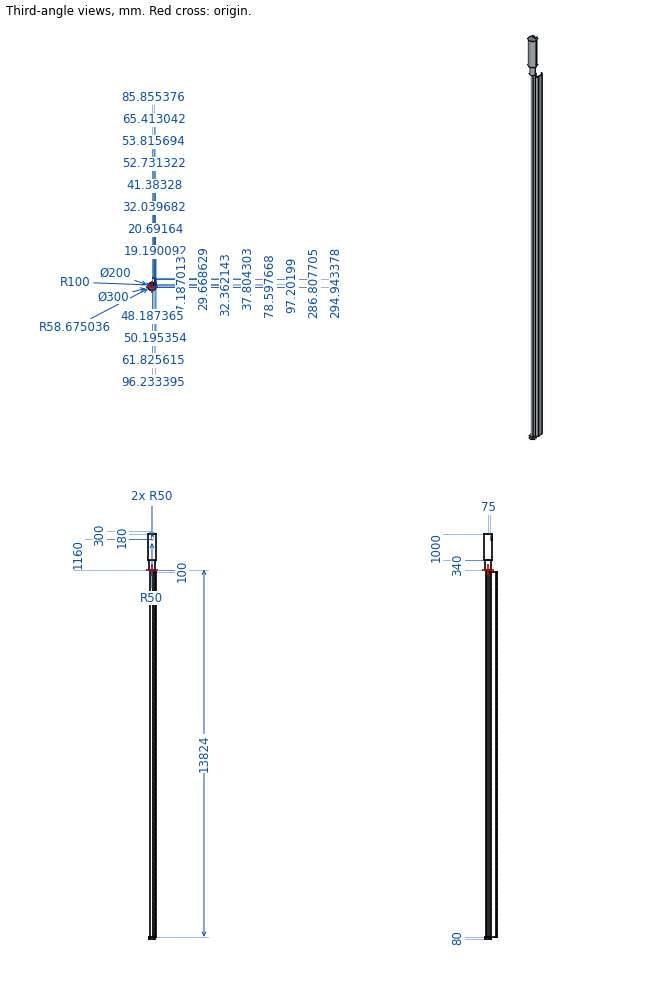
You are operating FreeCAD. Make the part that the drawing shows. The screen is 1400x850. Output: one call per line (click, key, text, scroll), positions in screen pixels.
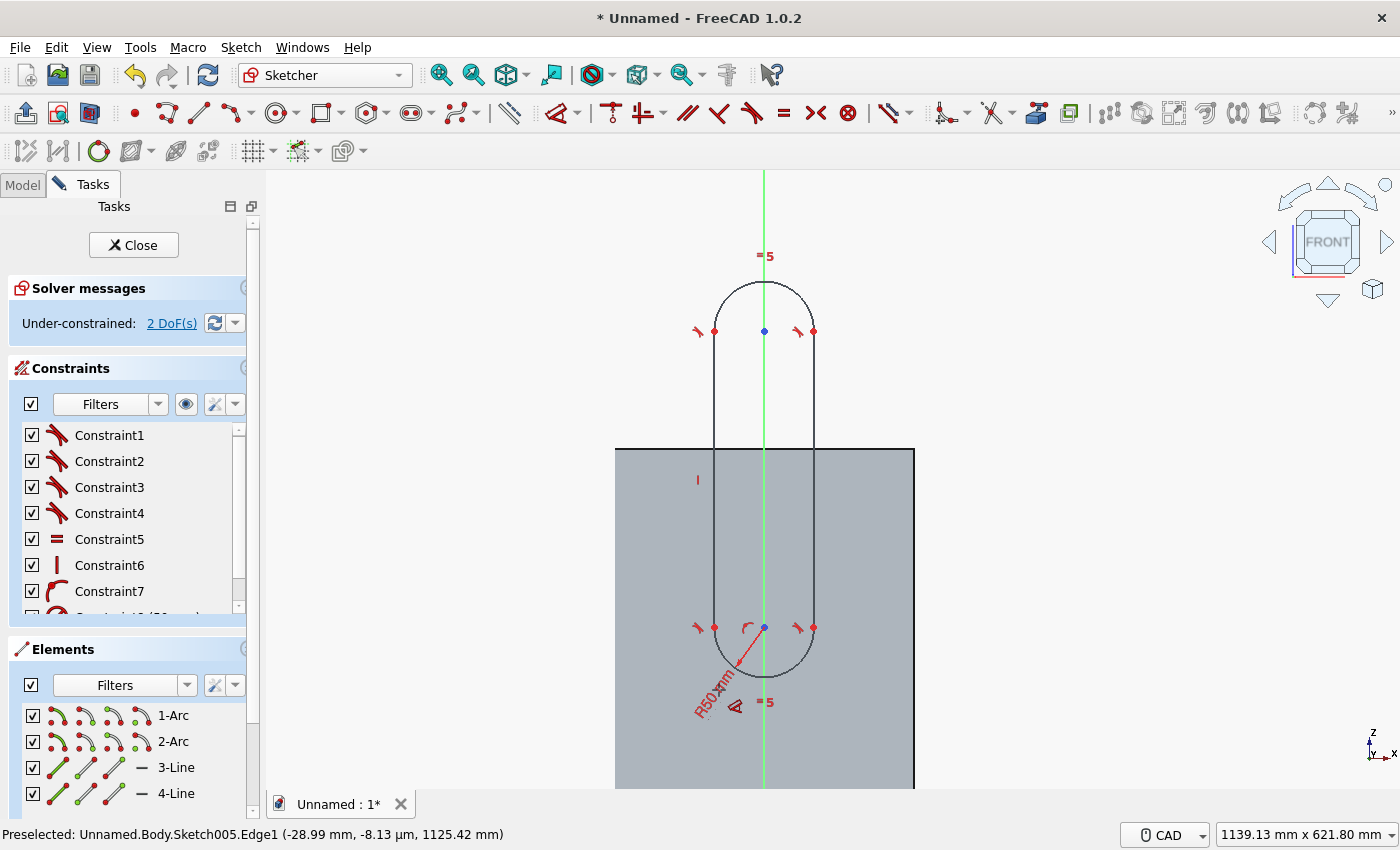
click(714, 539)
click(680, 479)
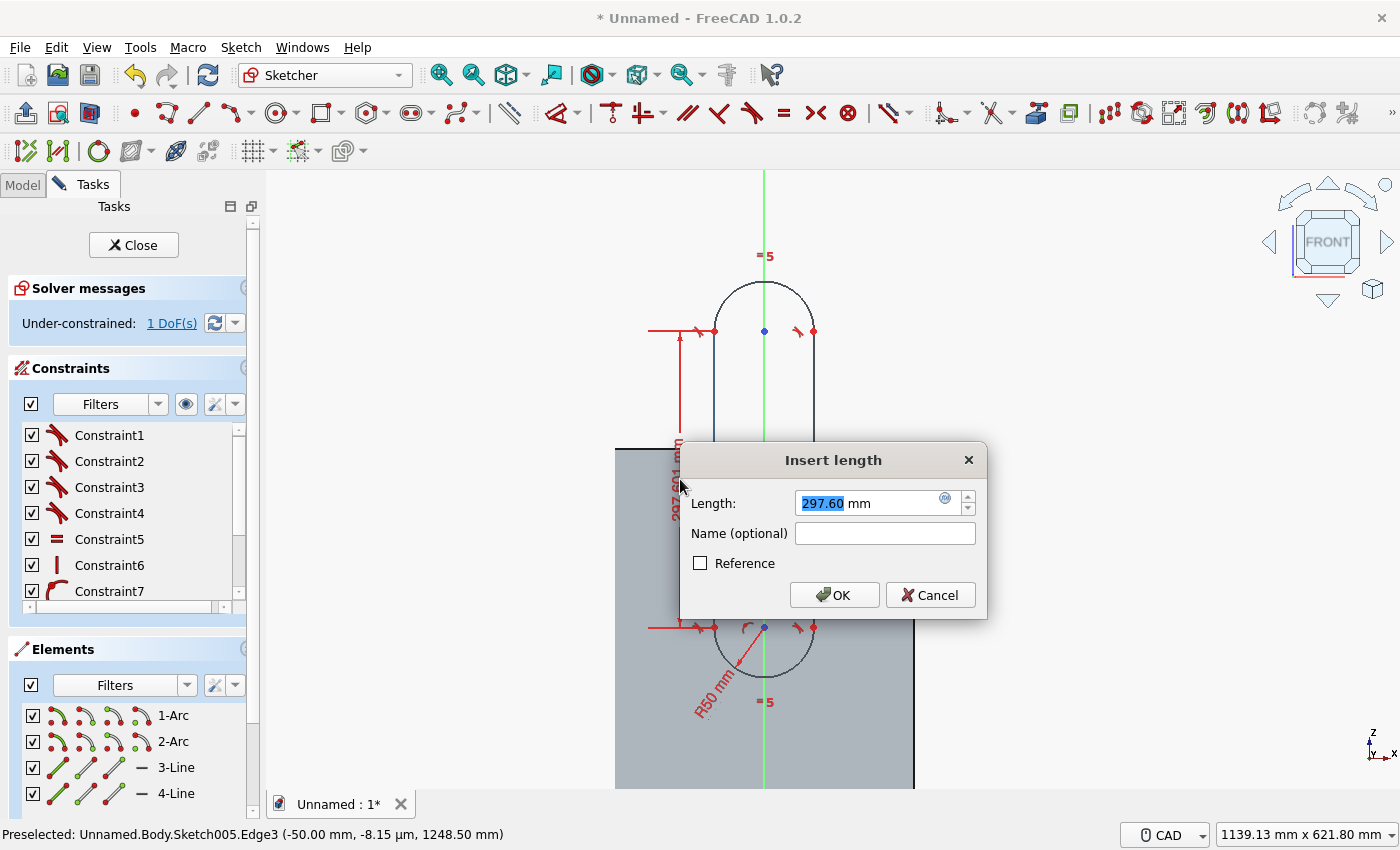
text(300)
key(Return)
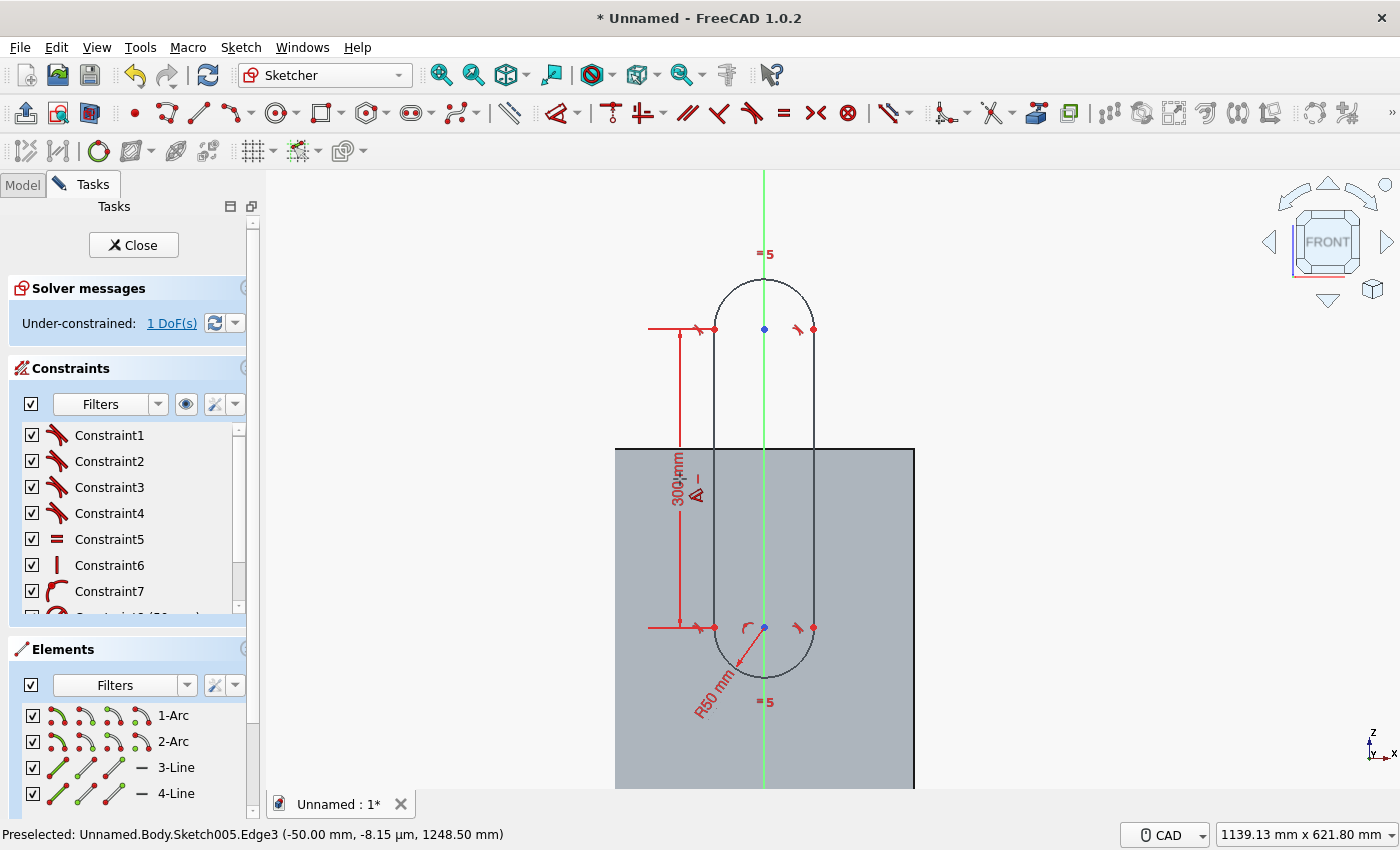
click(714, 628)
click(680, 664)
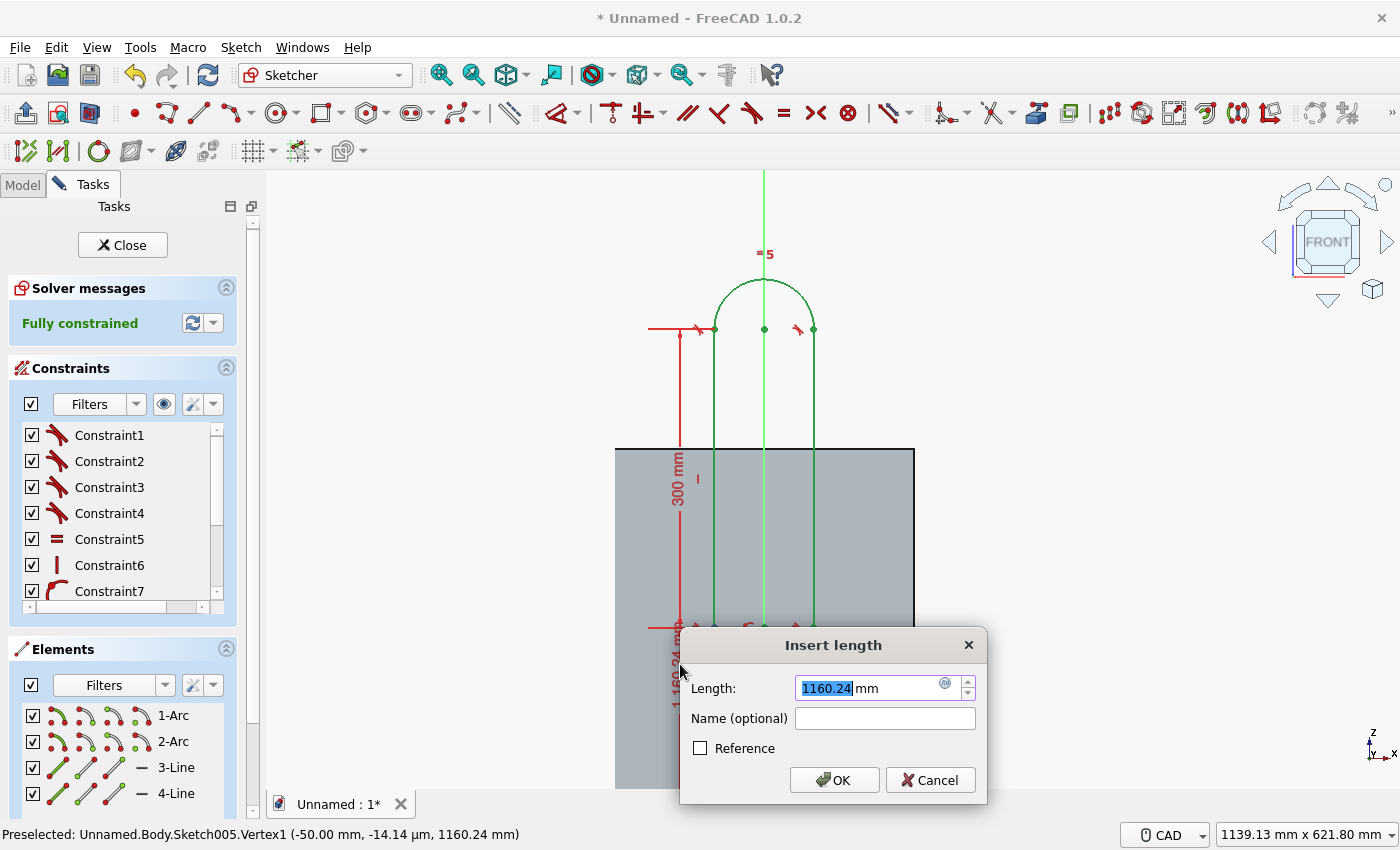
text(1160)
key(Return)
key(Escape)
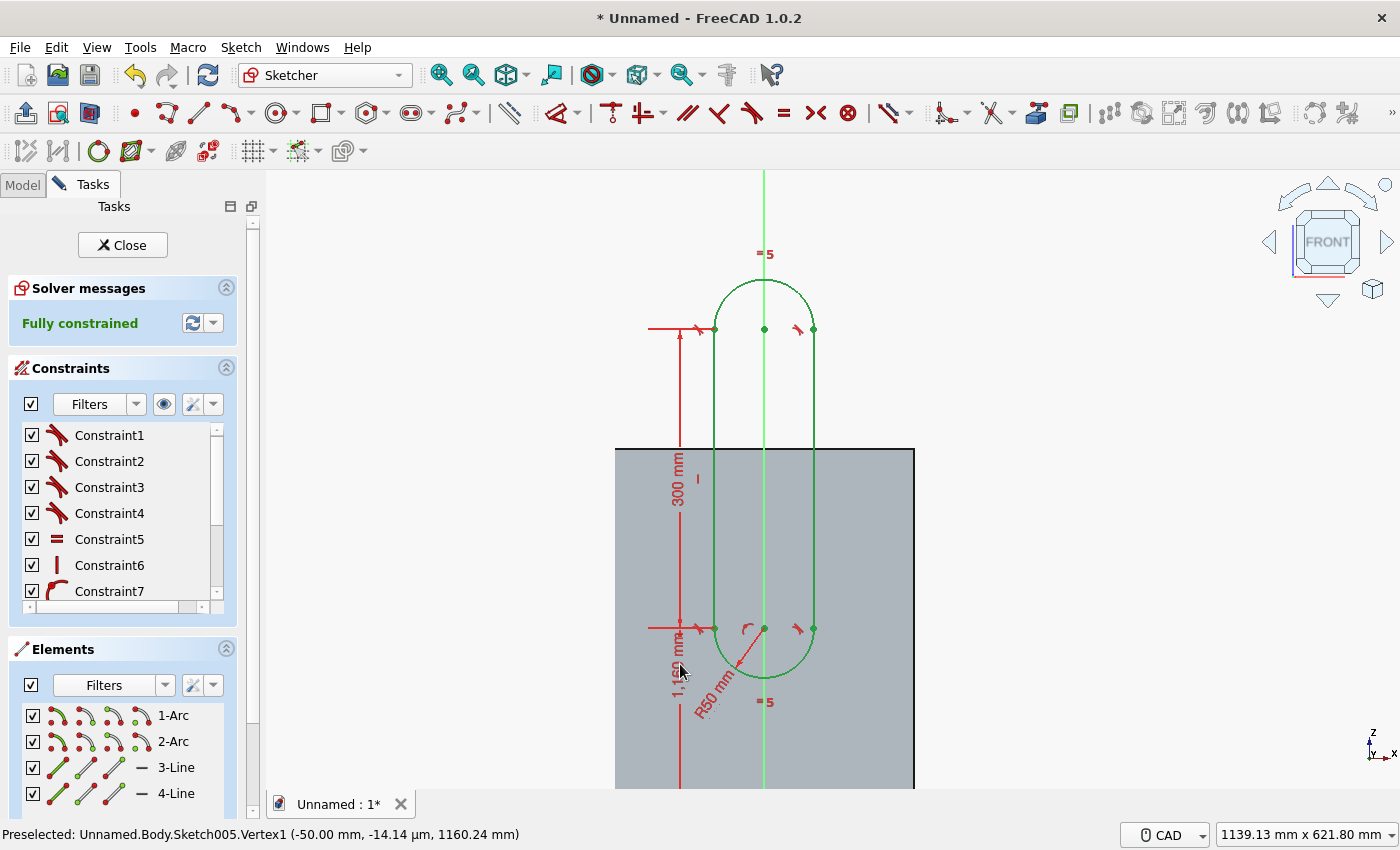
click(123, 245)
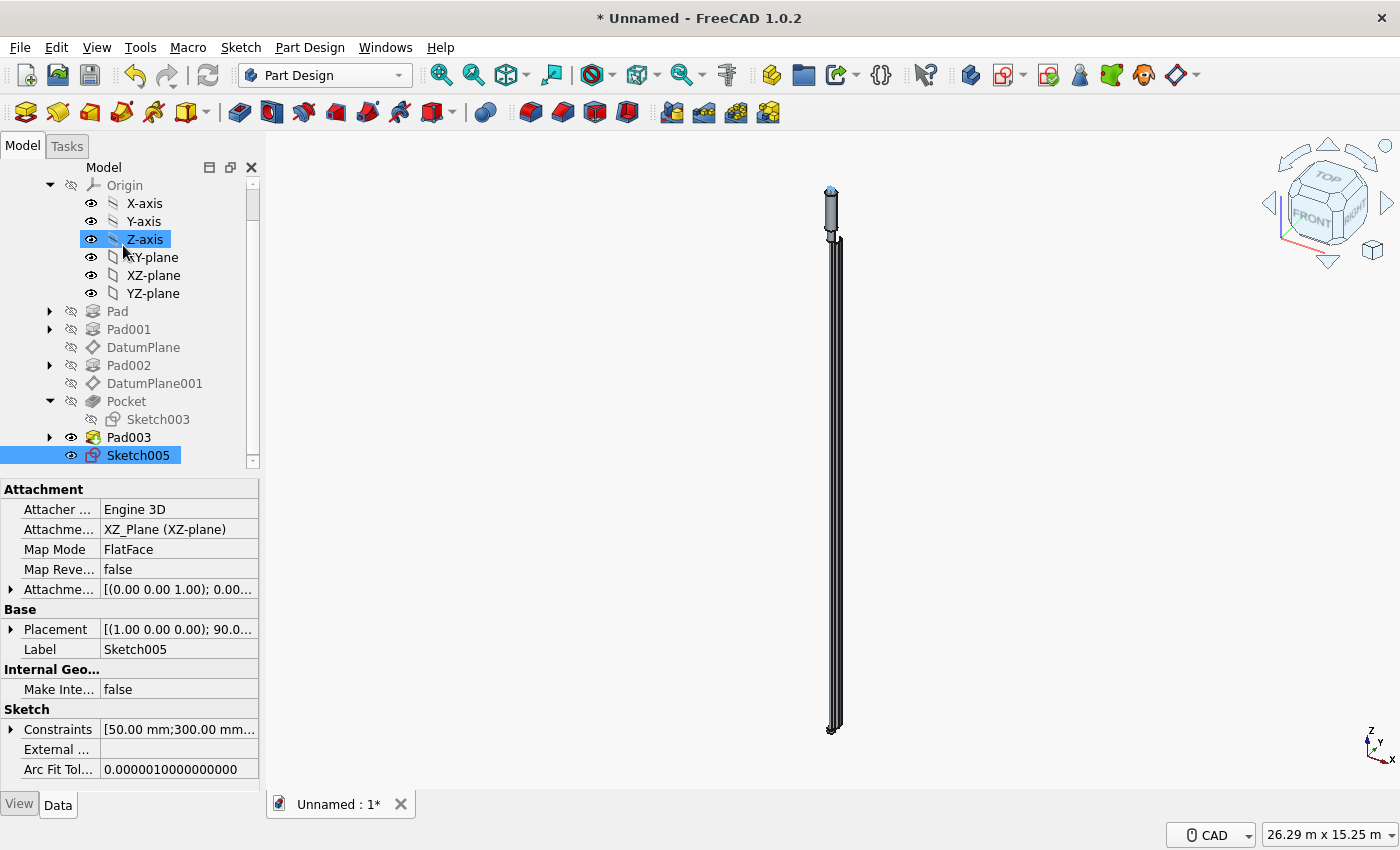
click(240, 112)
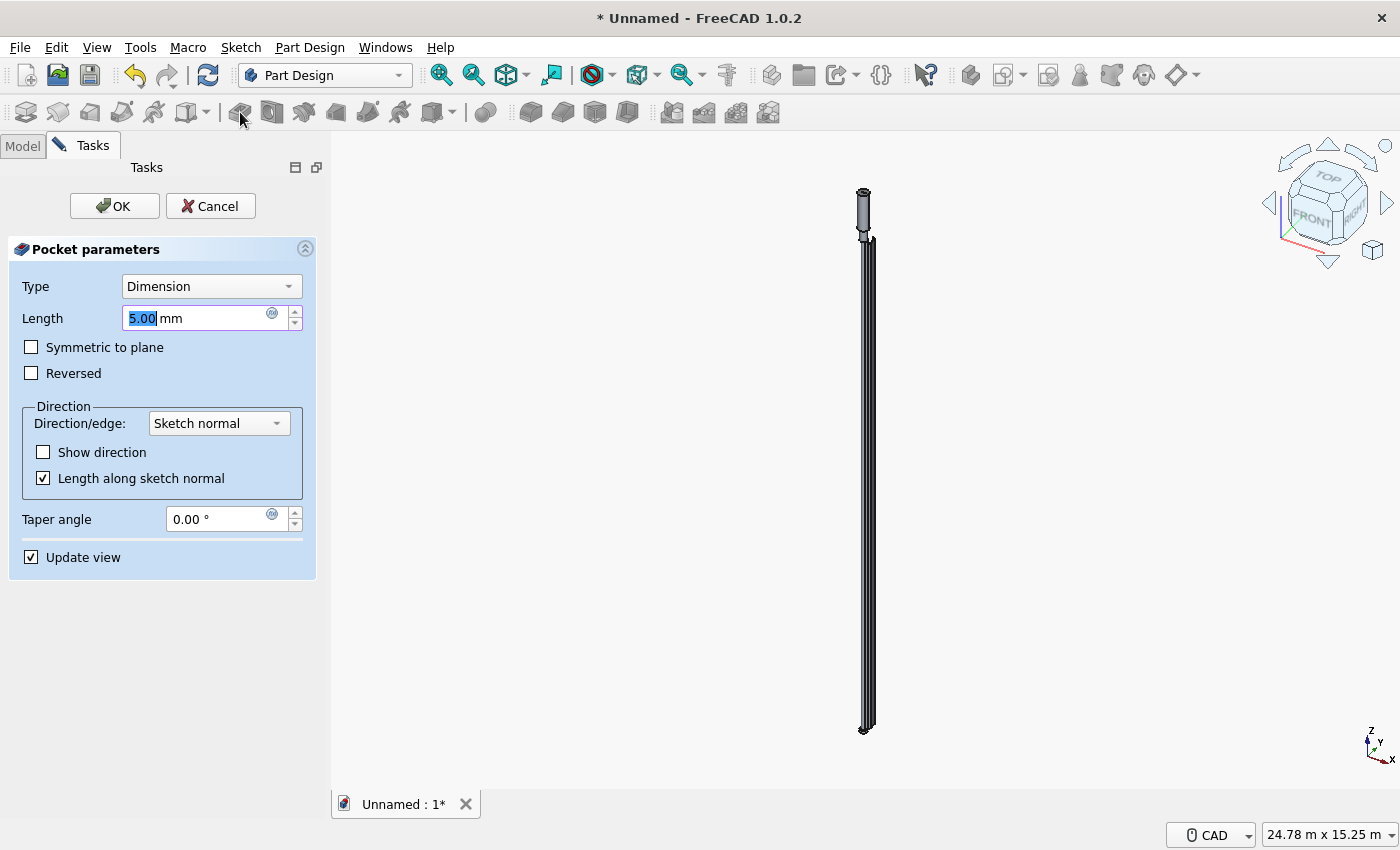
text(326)
key(Tab)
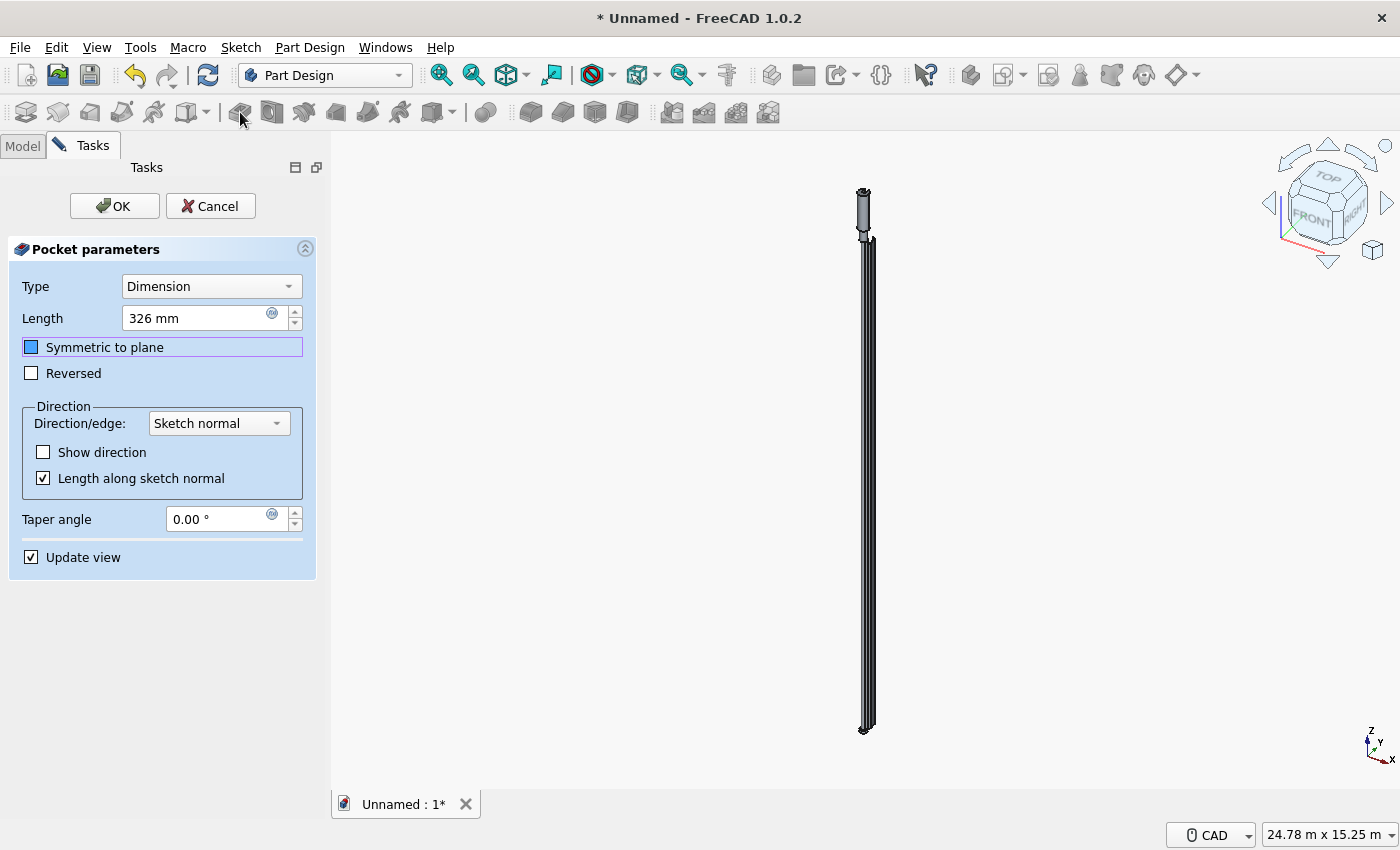
click(115, 206)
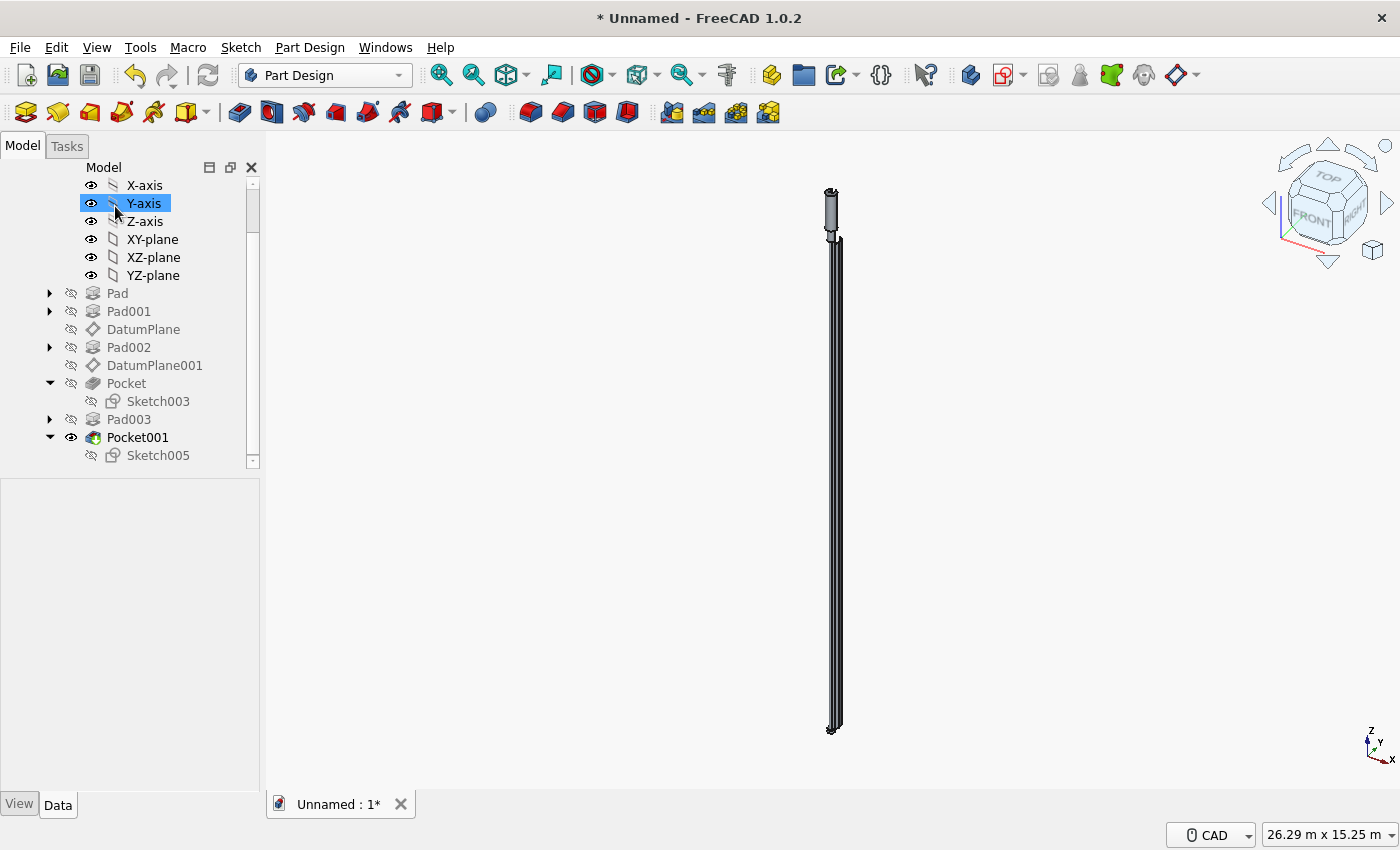
click(1004, 76)